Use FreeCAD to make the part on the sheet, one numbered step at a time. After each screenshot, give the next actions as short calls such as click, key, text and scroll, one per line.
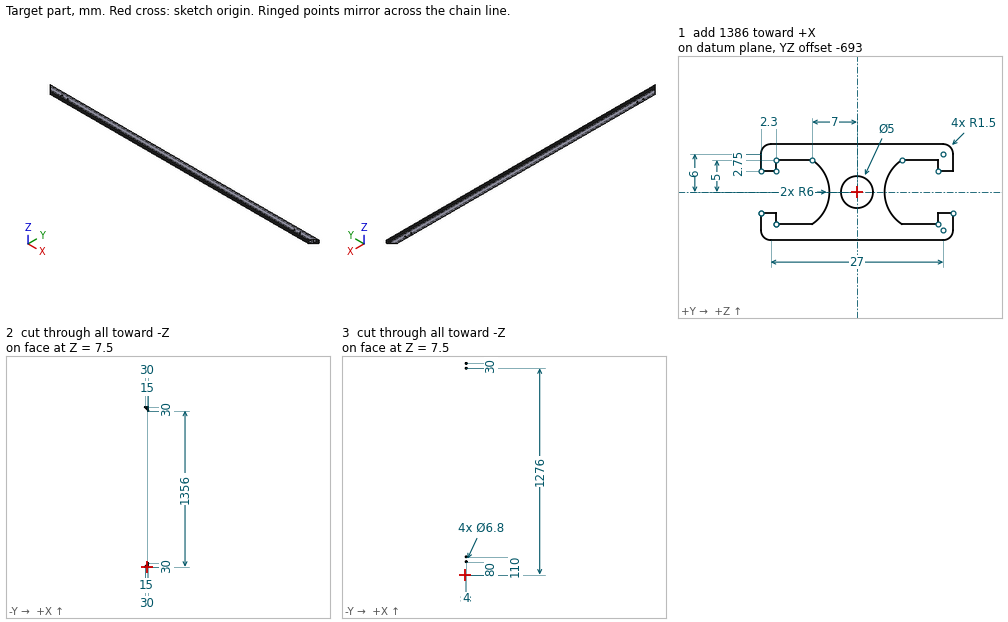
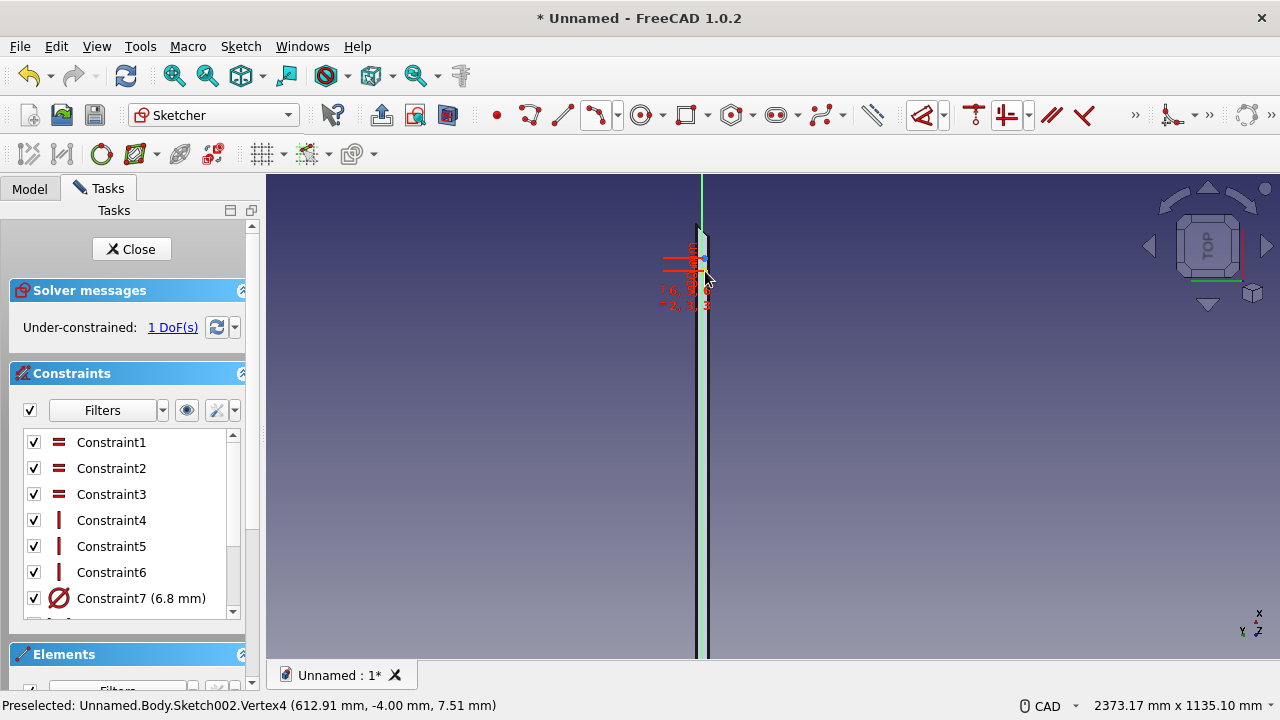
click(704, 271)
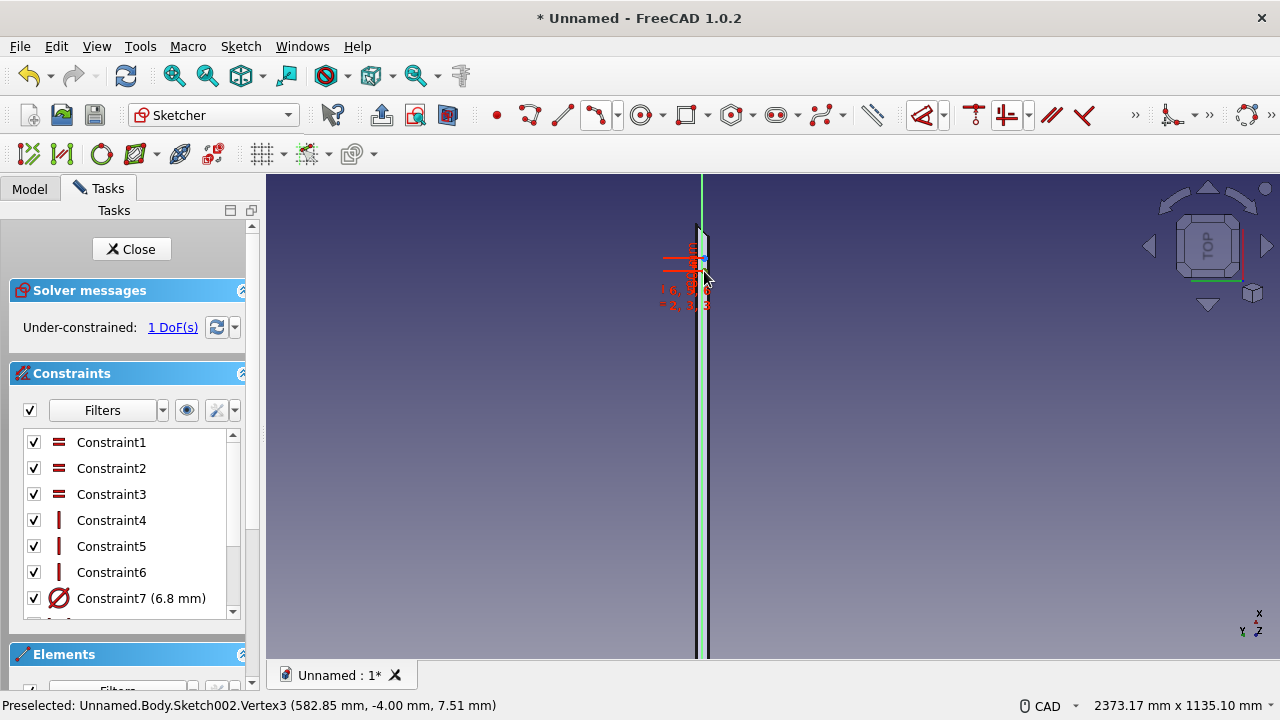
key(i)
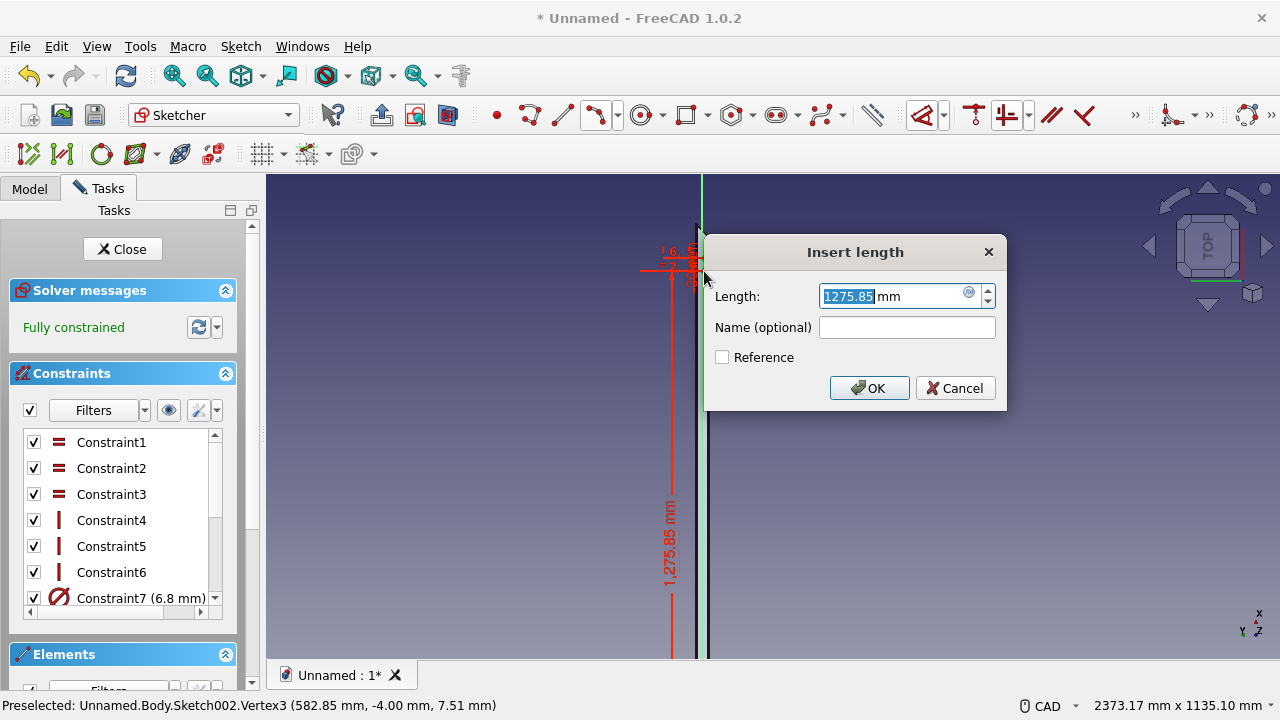
text(1276)
key(Return)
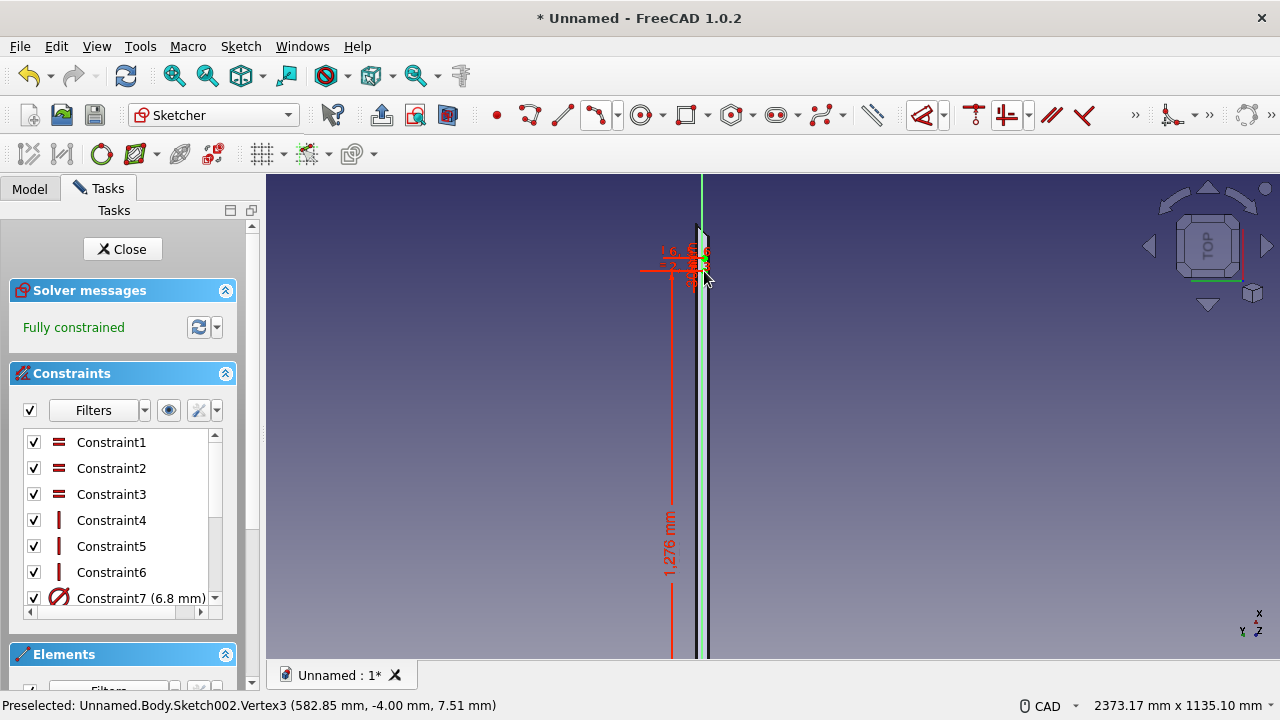
click(123, 249)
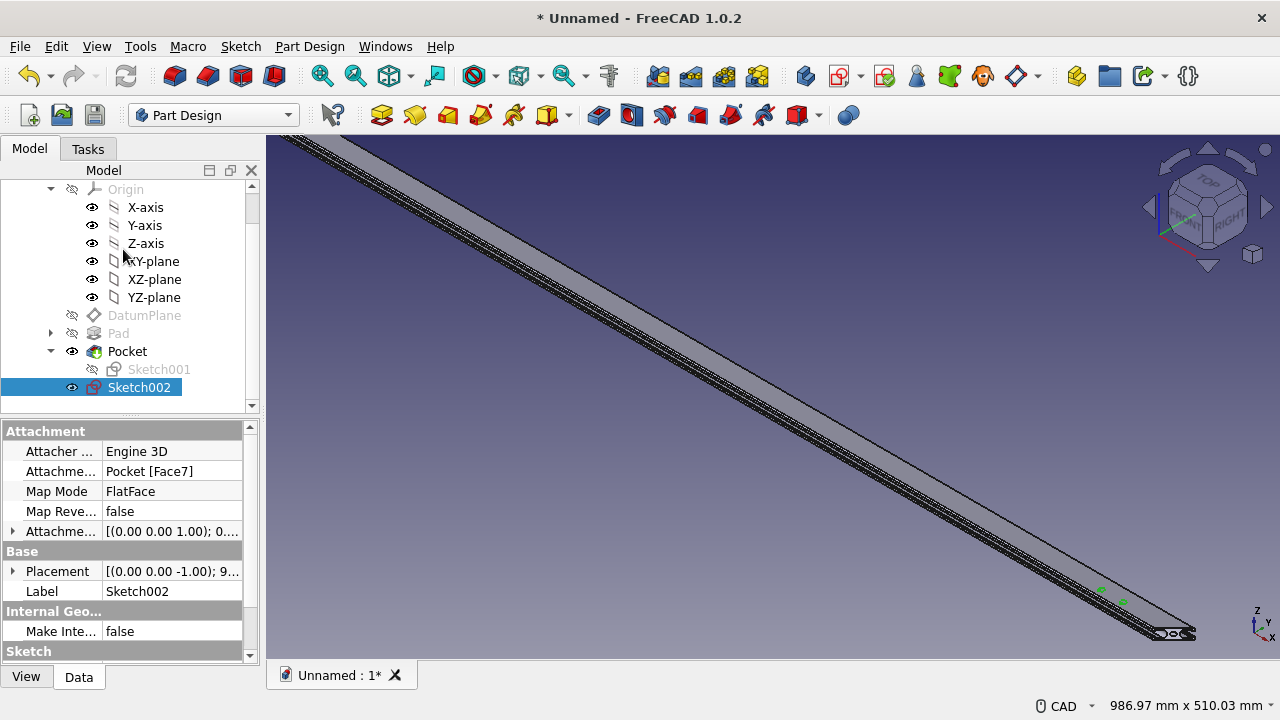
click(599, 116)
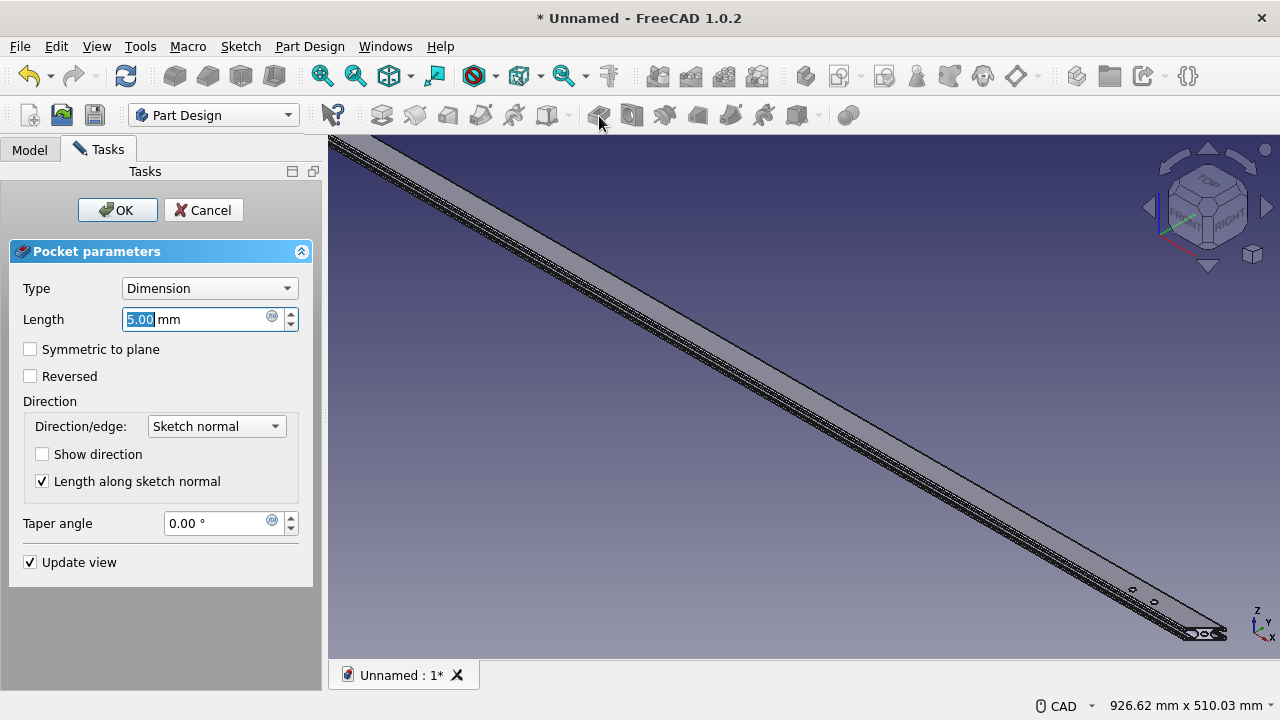
click(210, 288)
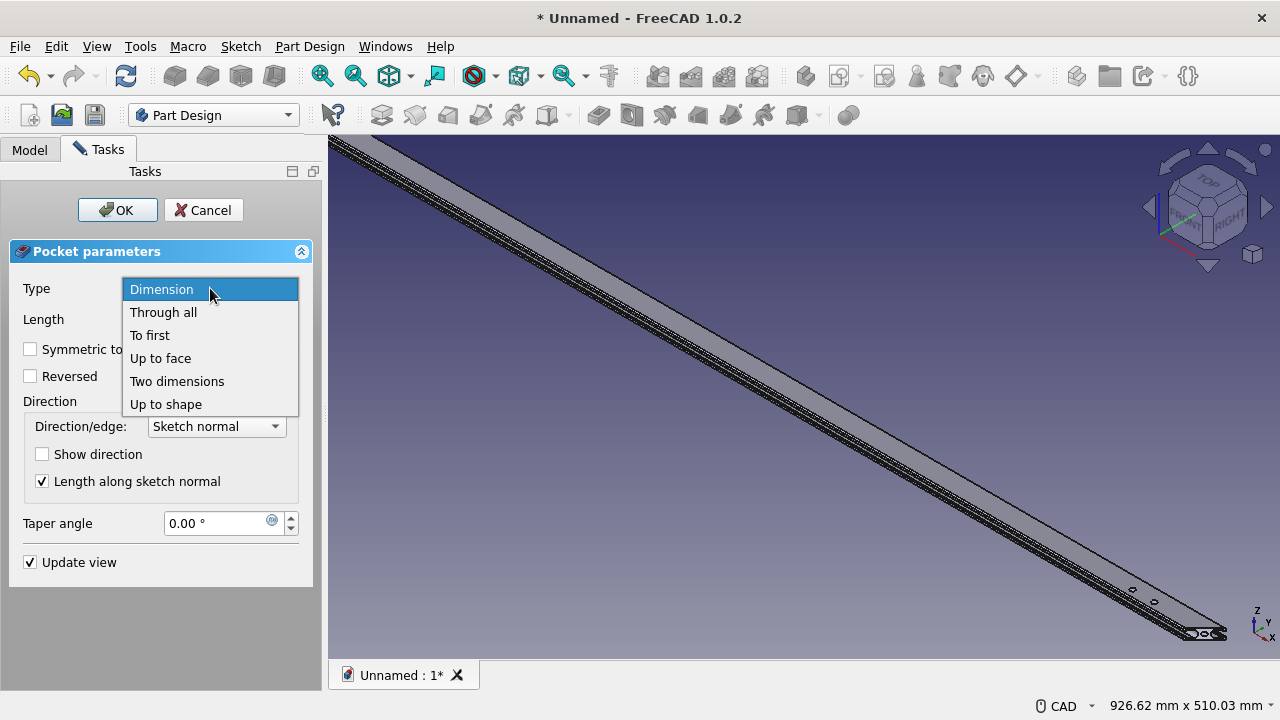
click(208, 312)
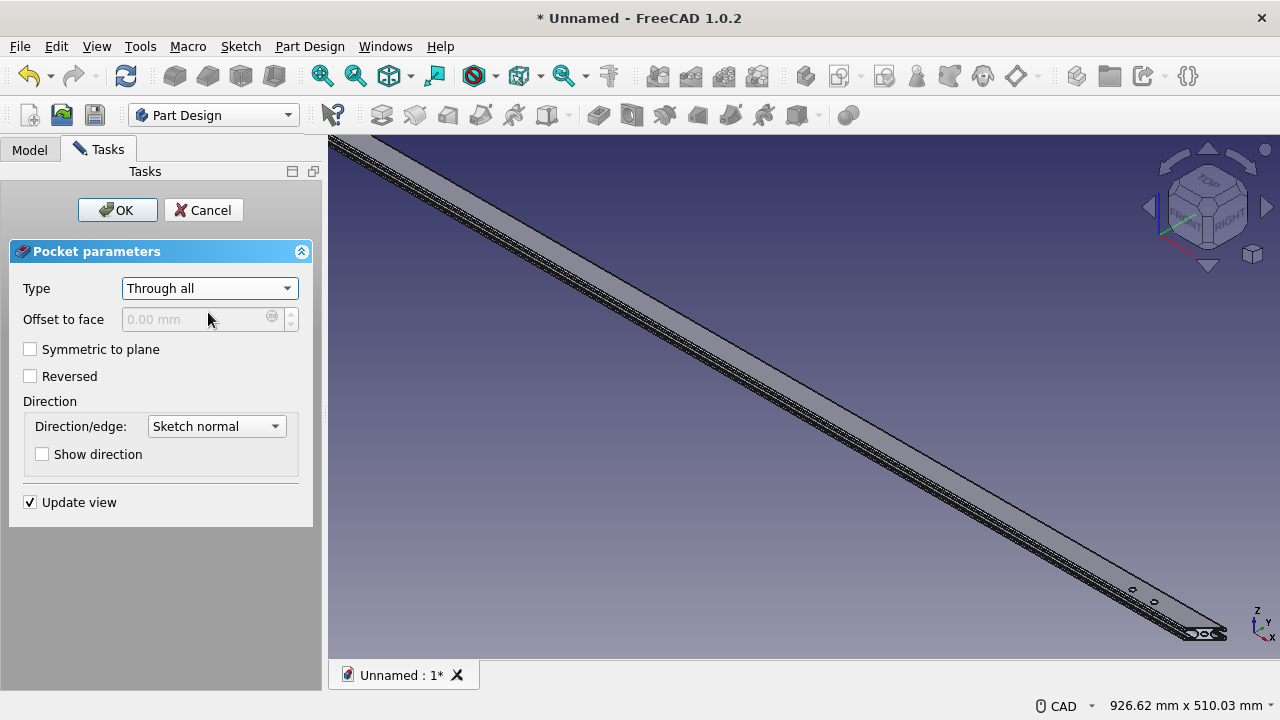
click(118, 210)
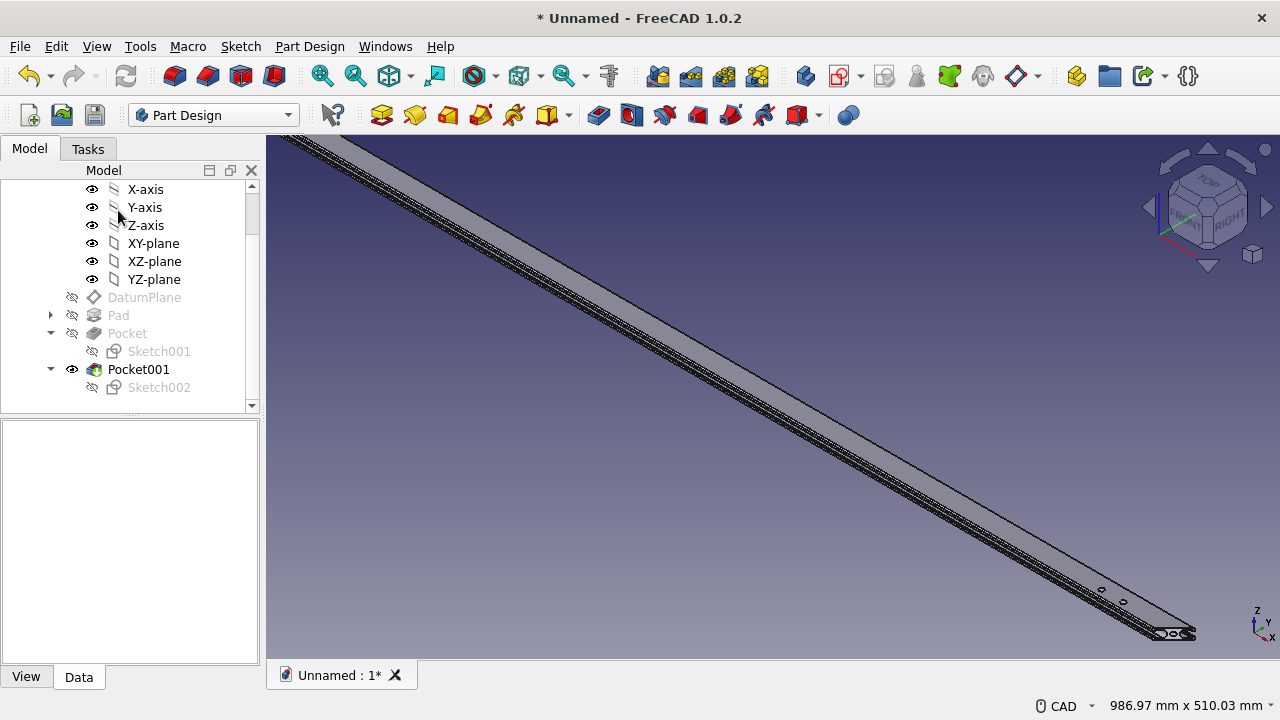
click(323, 76)